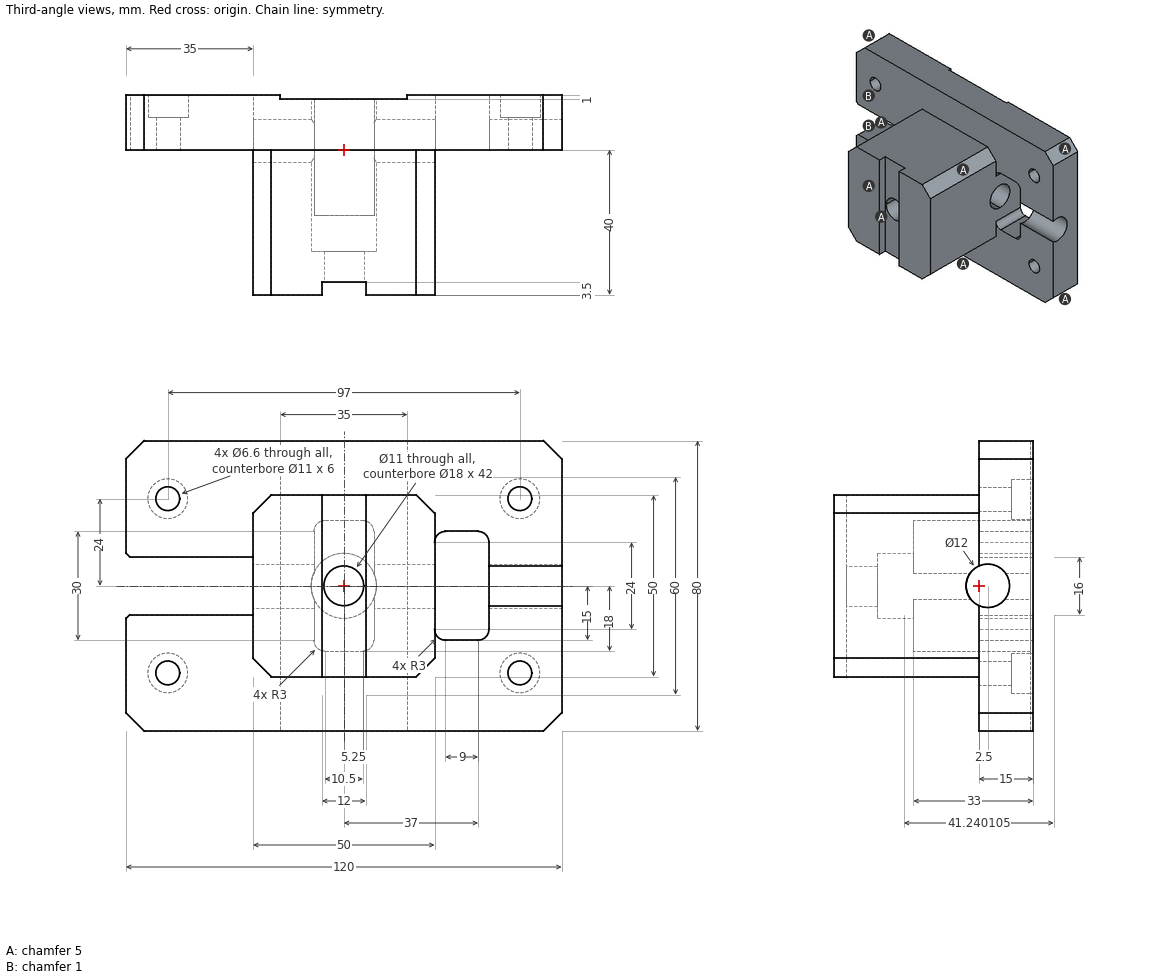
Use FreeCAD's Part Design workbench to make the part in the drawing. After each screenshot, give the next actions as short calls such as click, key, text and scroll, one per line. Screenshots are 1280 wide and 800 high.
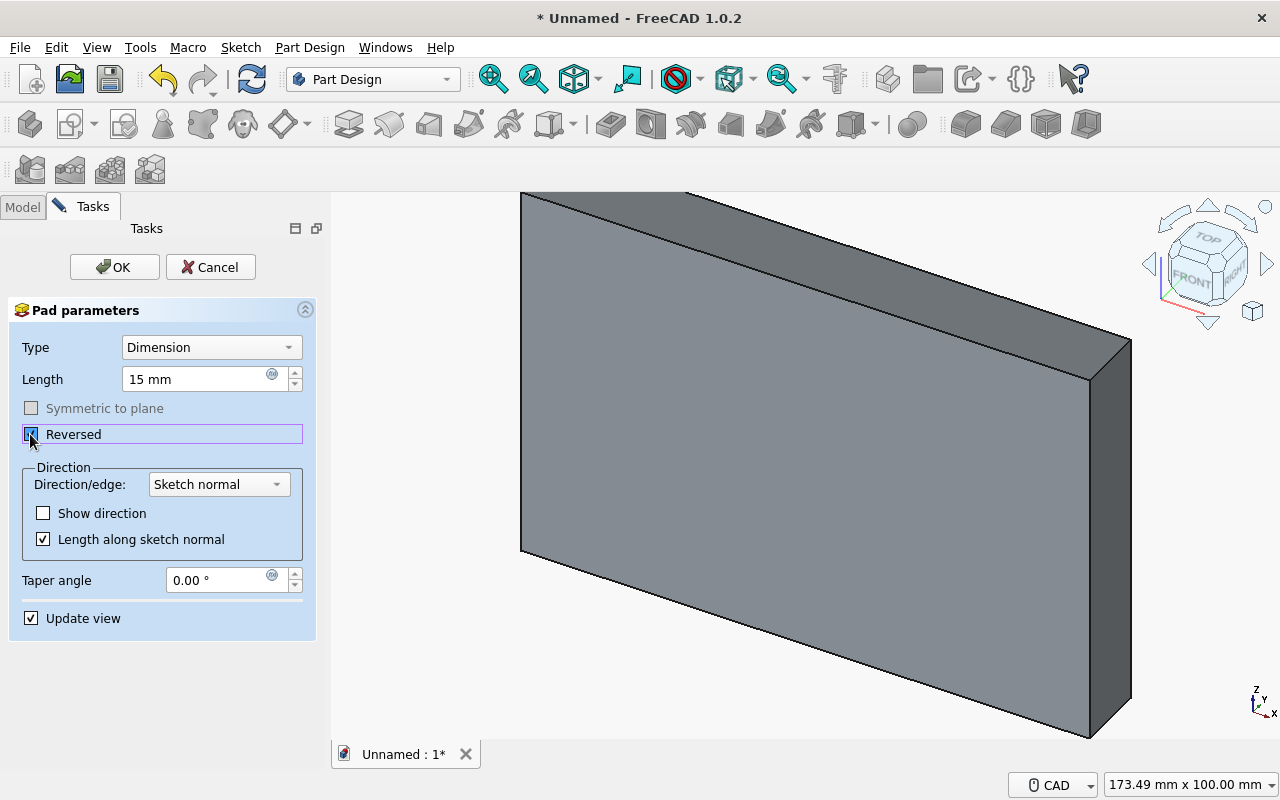
click(115, 267)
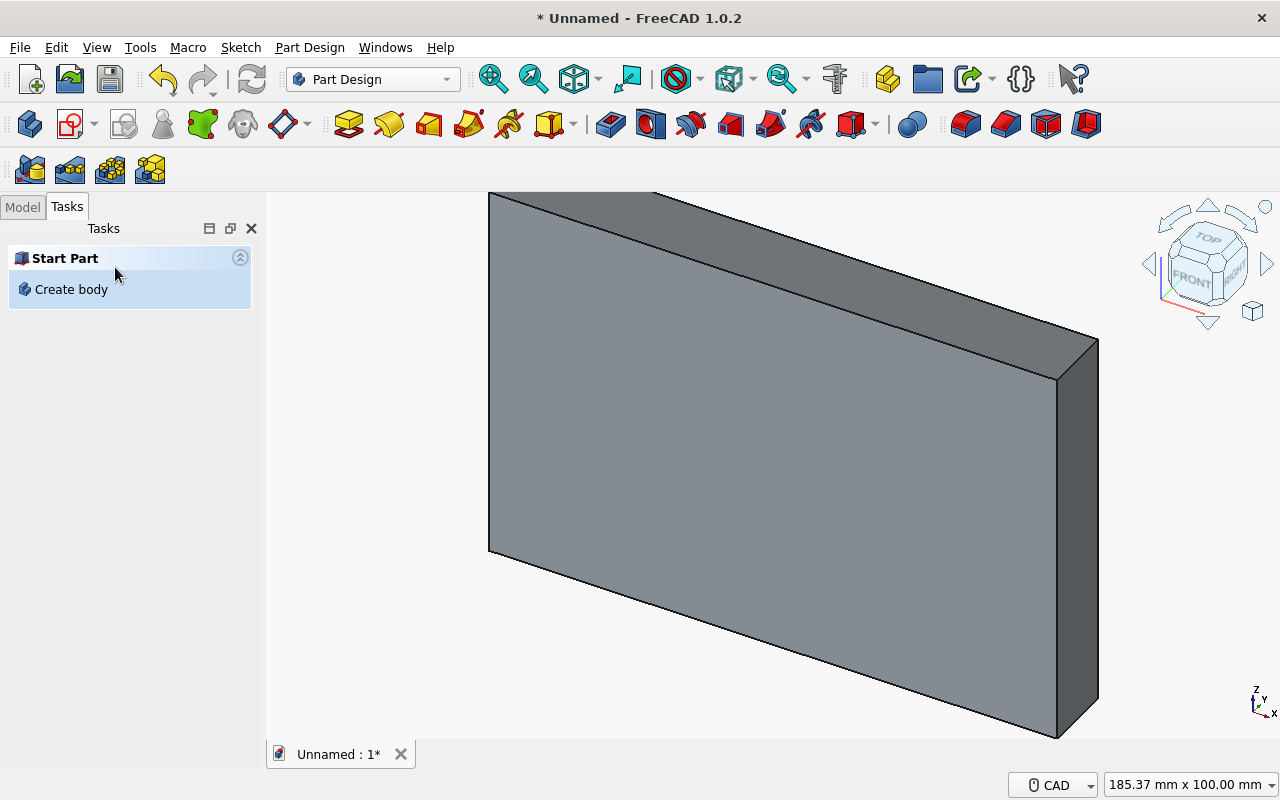
key(v)
key(f)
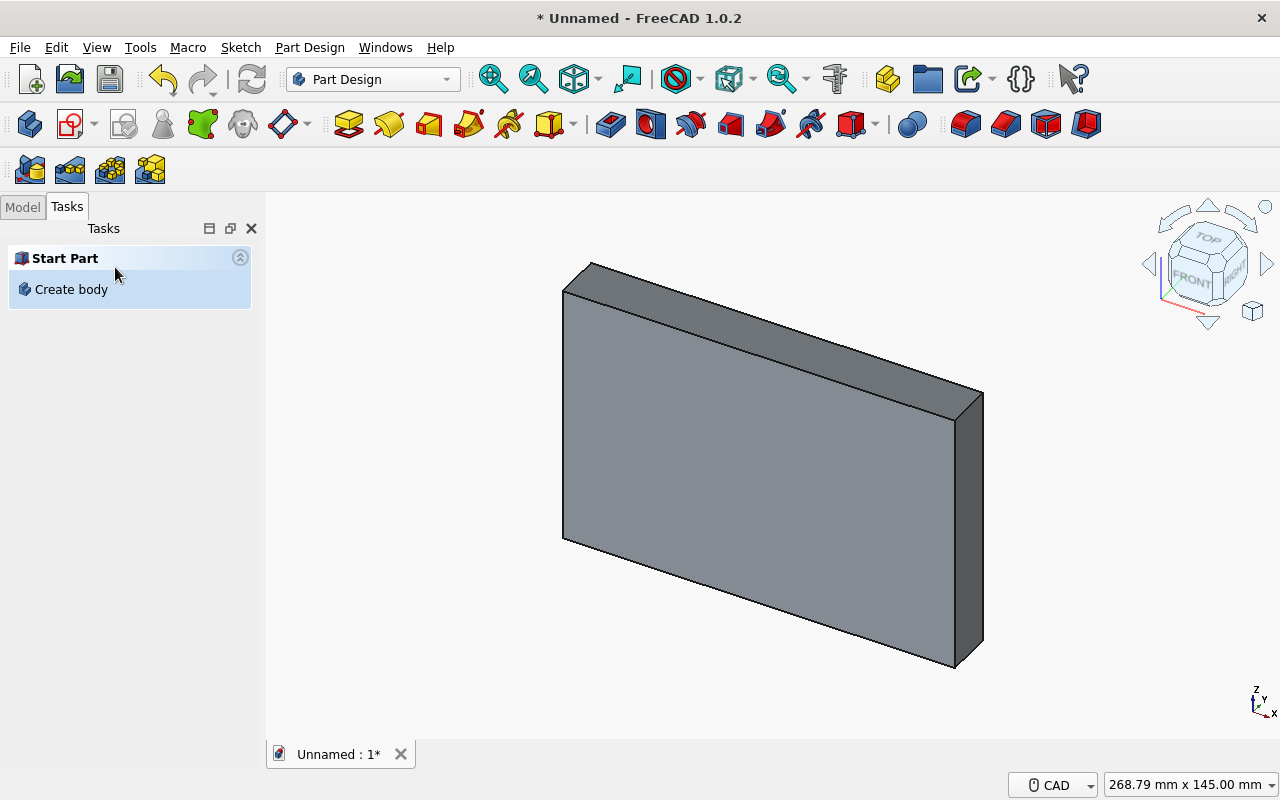
click(815, 497)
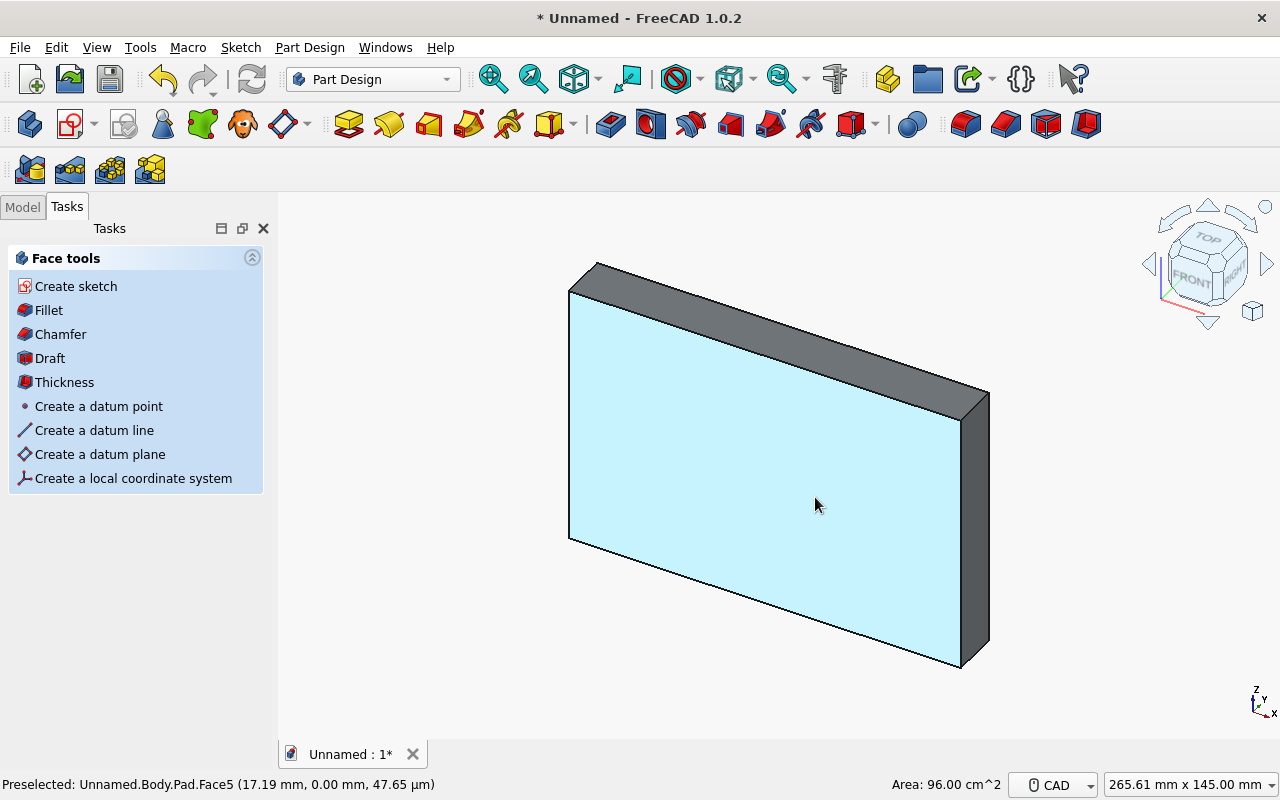
click(70, 124)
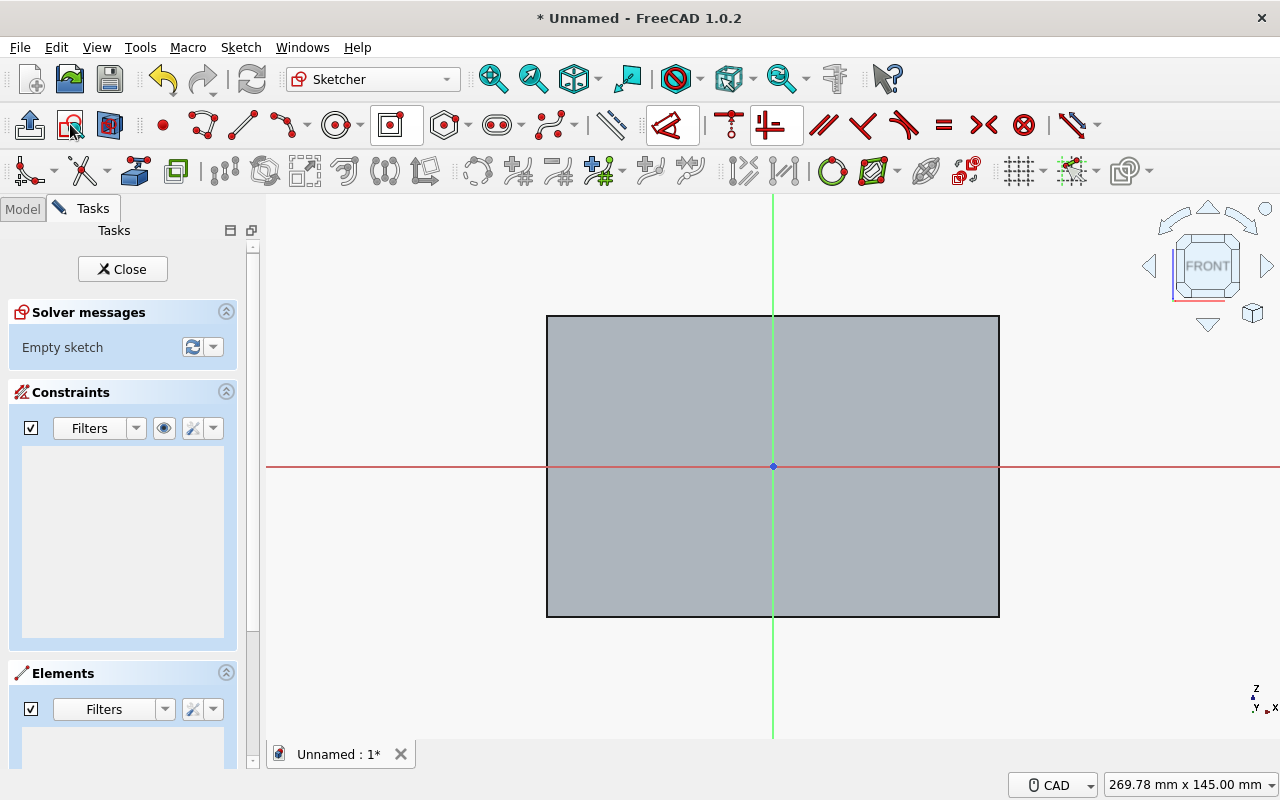
scroll(856, 467, up, 3)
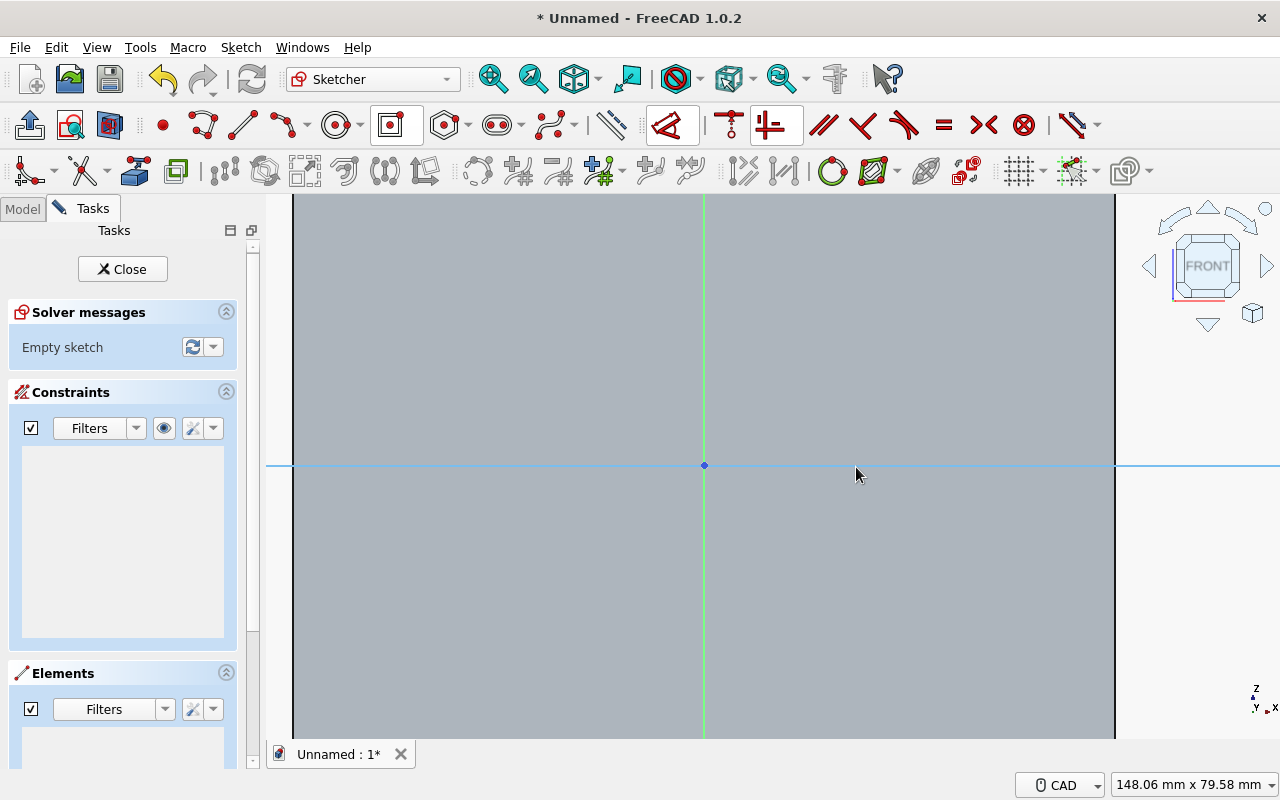
click(390, 126)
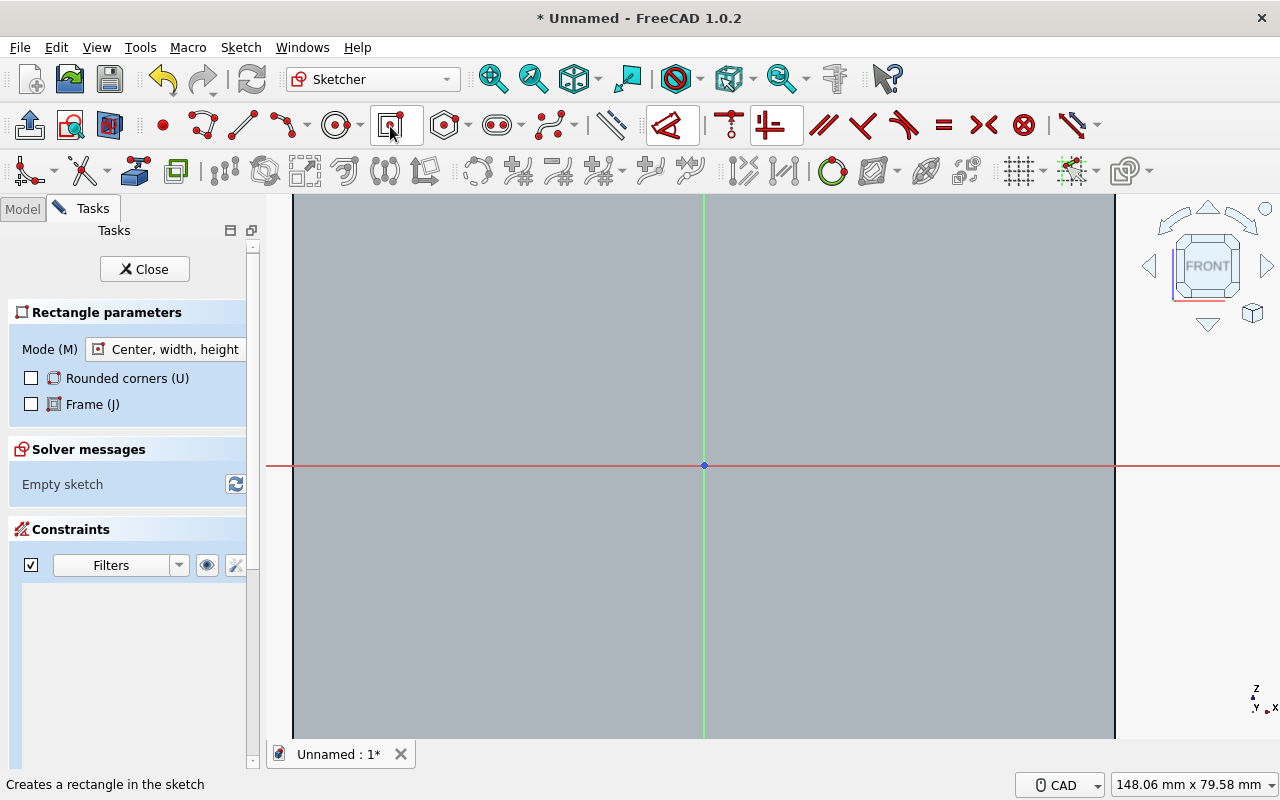
click(704, 466)
click(876, 294)
key(Escape)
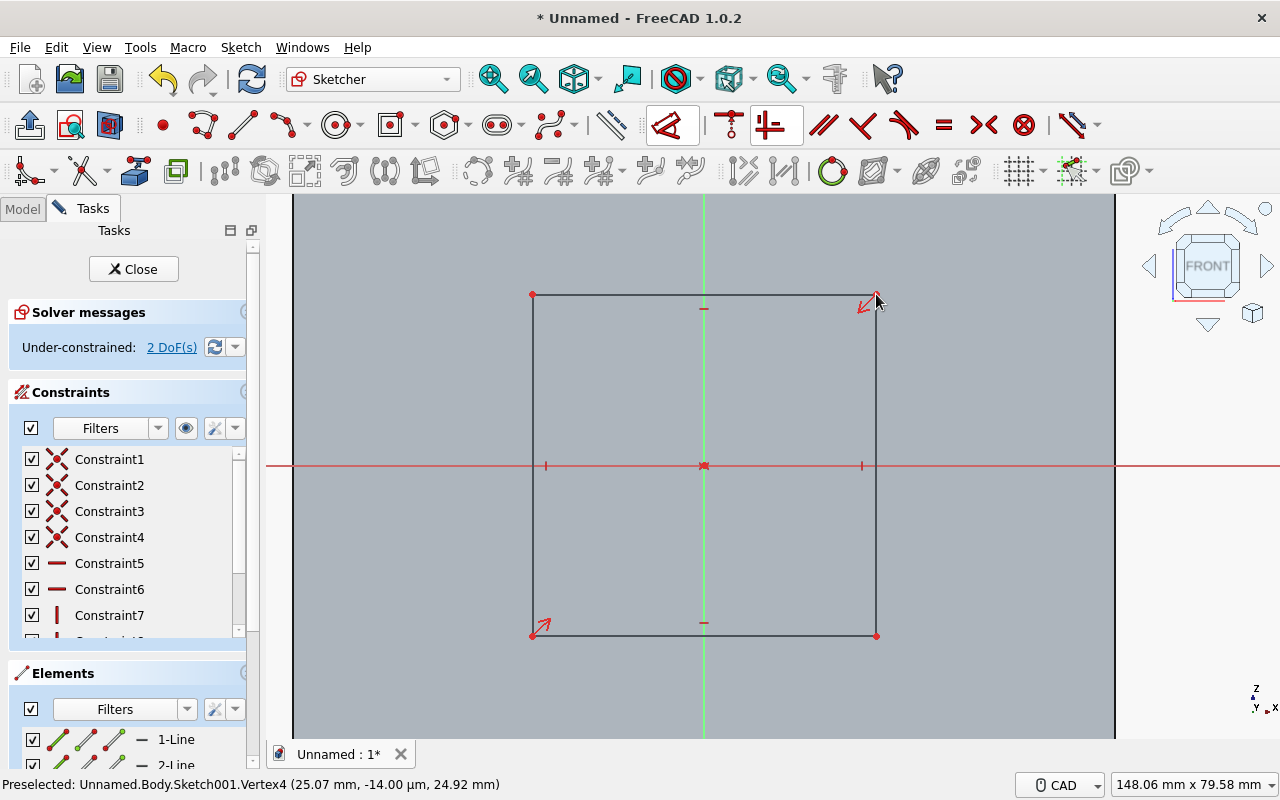
click(636, 636)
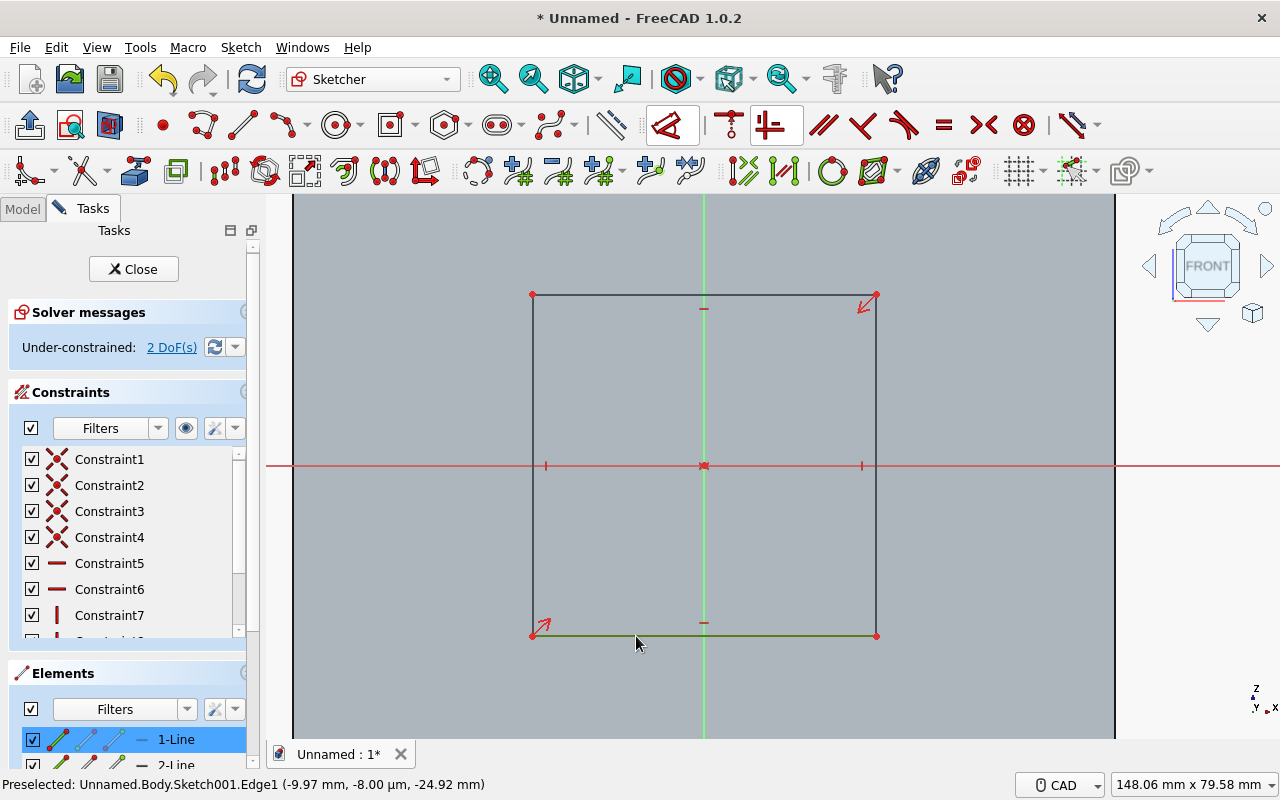
click(694, 126)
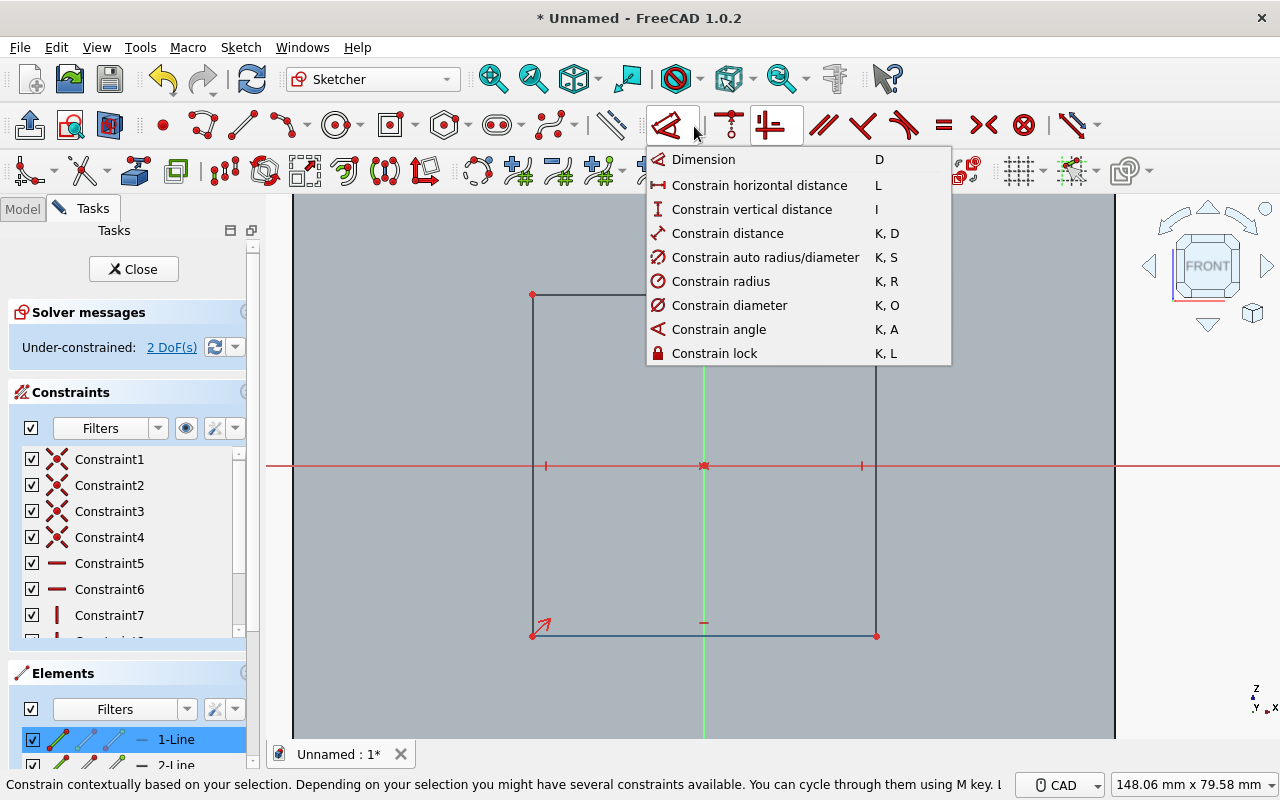
click(799, 185)